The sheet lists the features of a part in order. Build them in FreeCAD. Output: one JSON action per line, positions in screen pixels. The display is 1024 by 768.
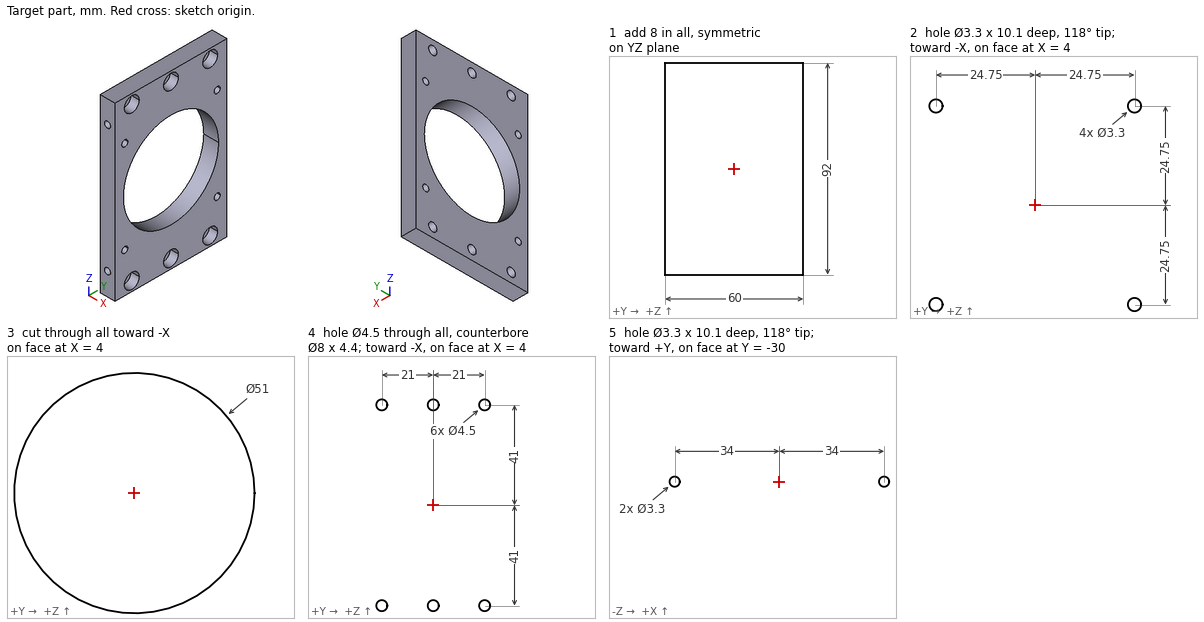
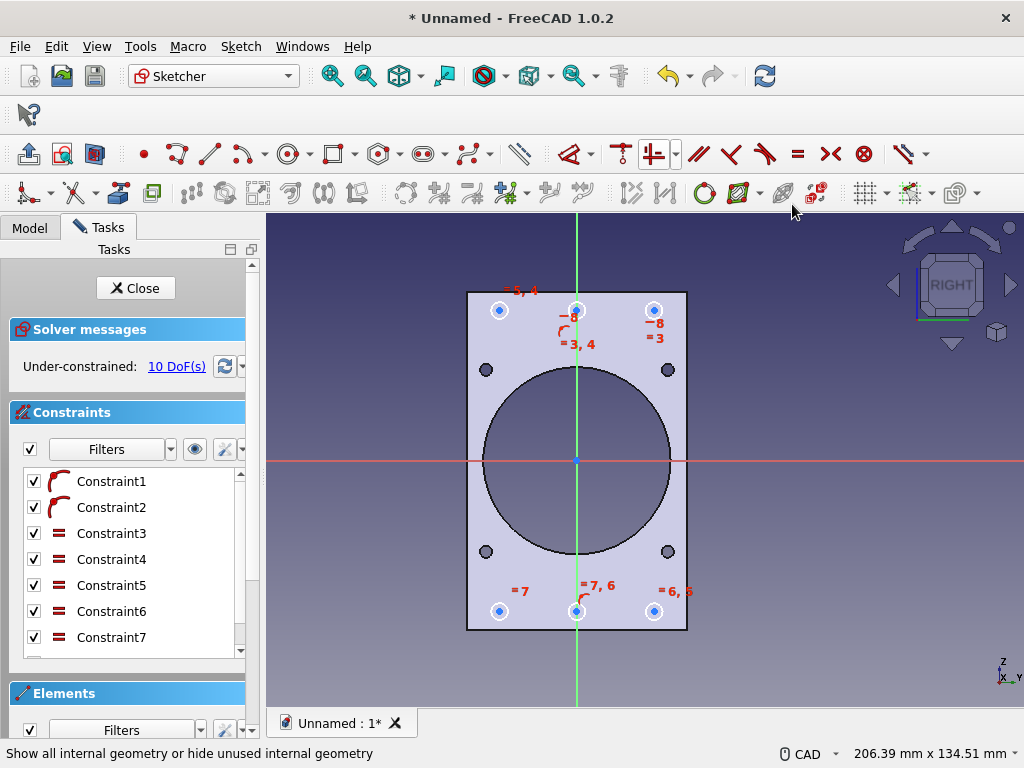
{"action": "scroll", "coordinate": [577, 311], "scroll_direction": "up", "scroll_amount": 4}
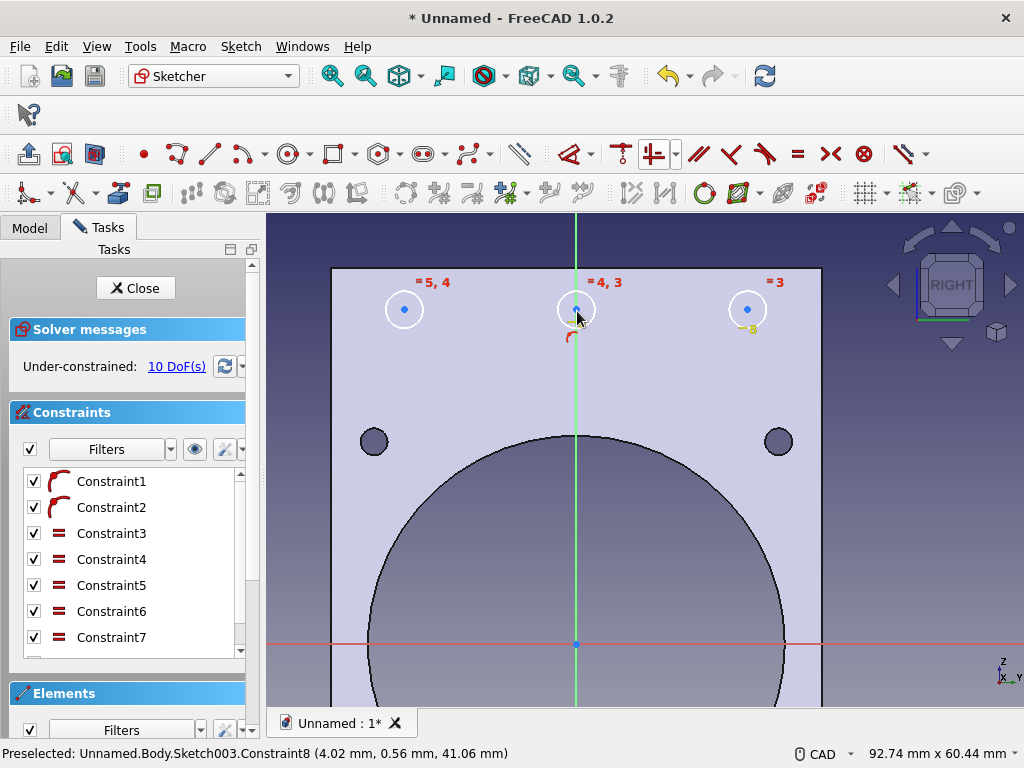
{"action": "left_click", "coordinate": [576, 310]}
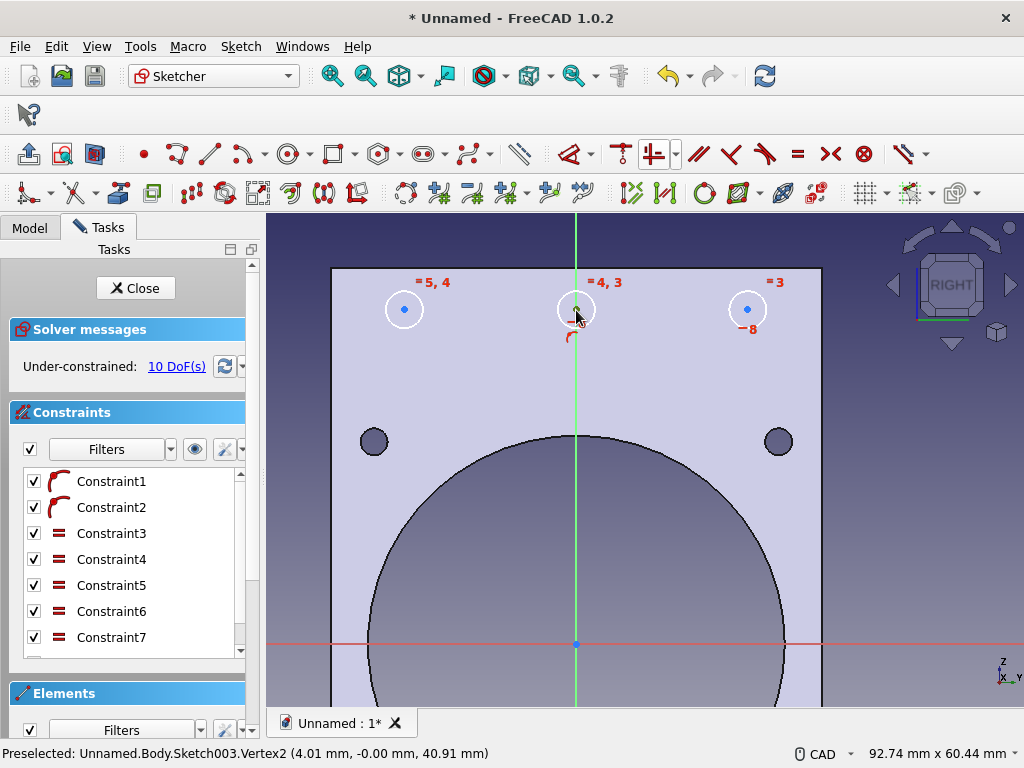
{"action": "left_click", "coordinate": [404, 310]}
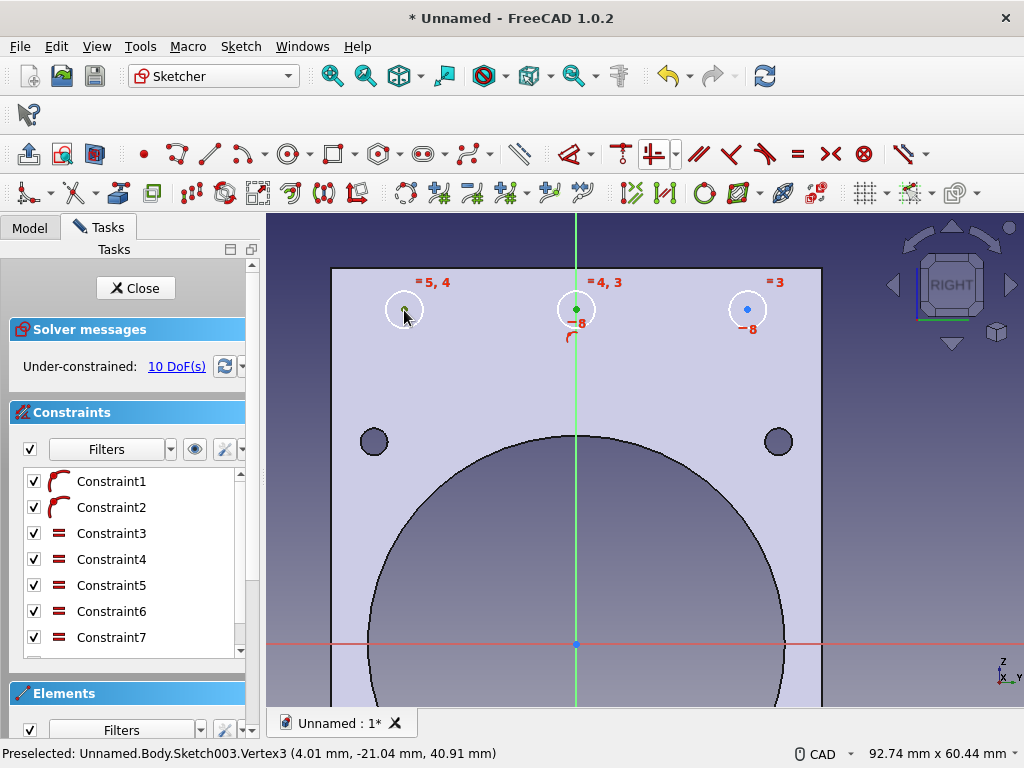
{"action": "left_click", "coordinate": [676, 154]}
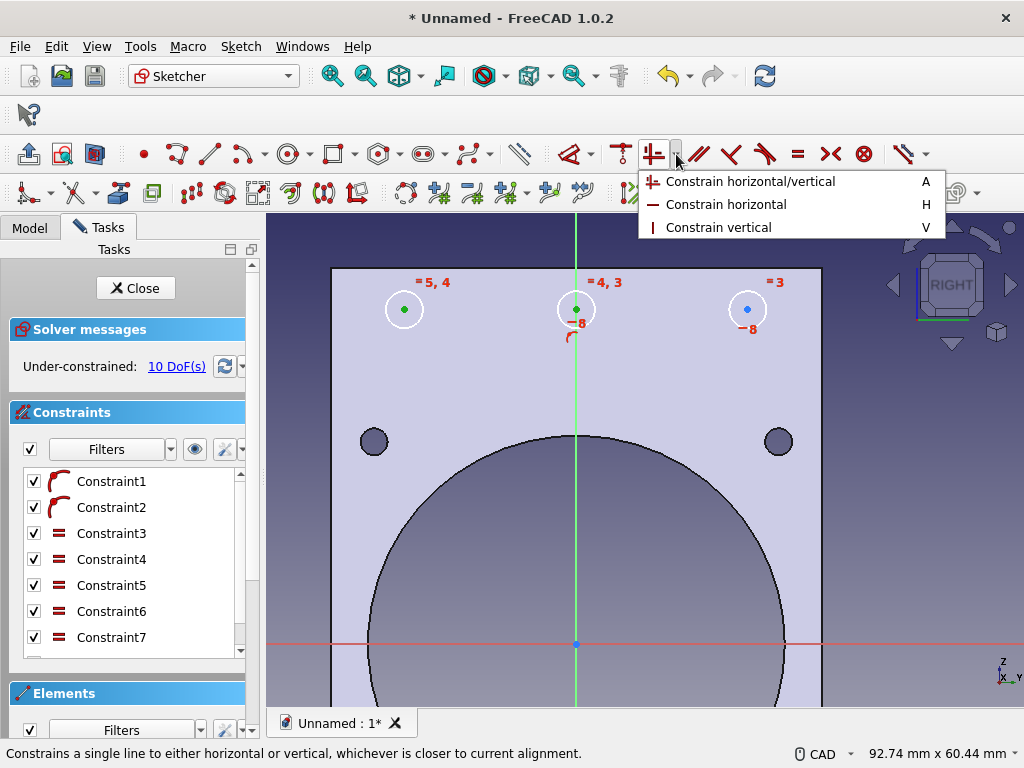
{"action": "left_click", "coordinate": [792, 204]}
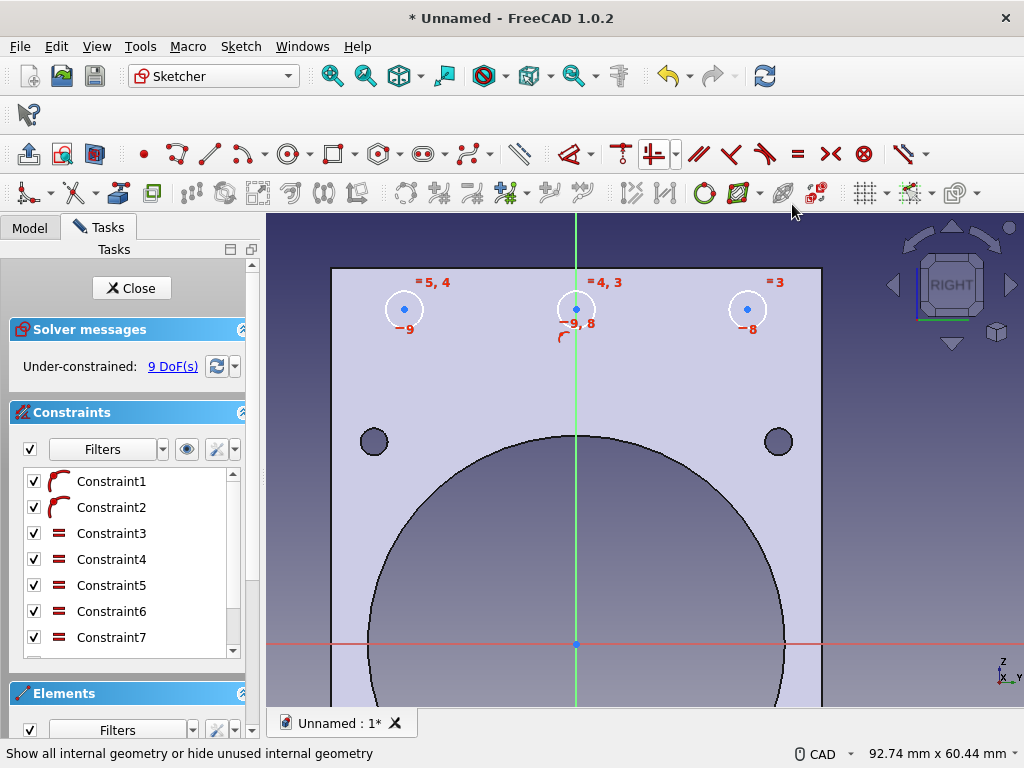
{"action": "left_click", "coordinate": [748, 310]}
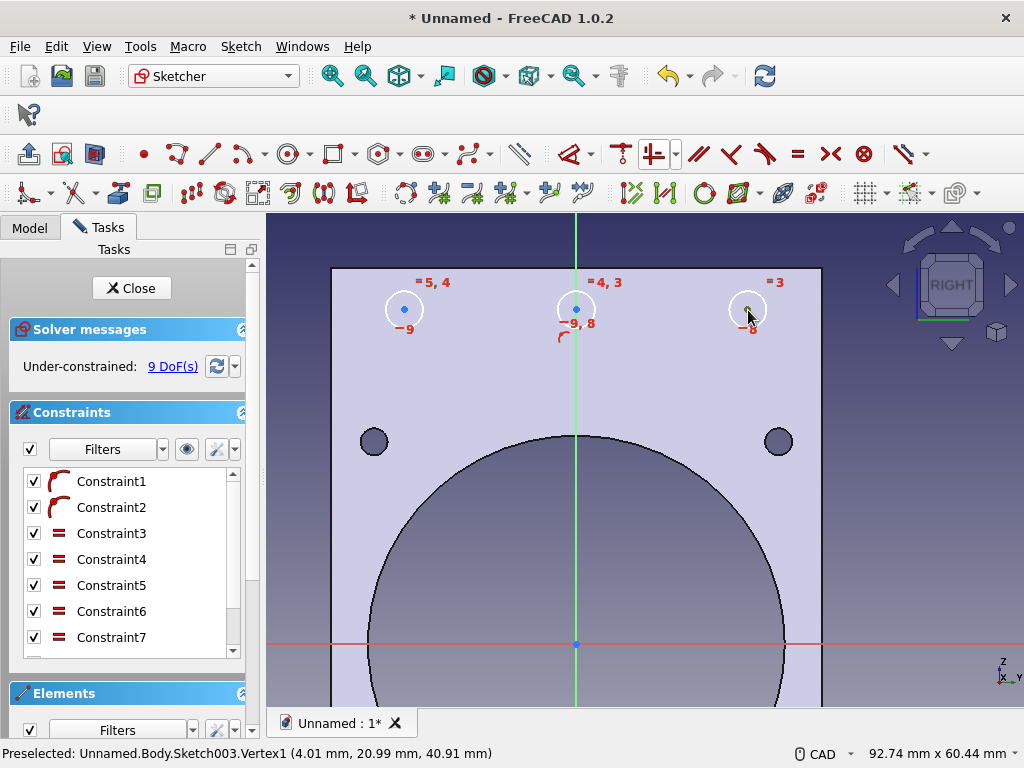
{"action": "scroll", "coordinate": [577, 310], "scroll_direction": "down", "scroll_amount": 4}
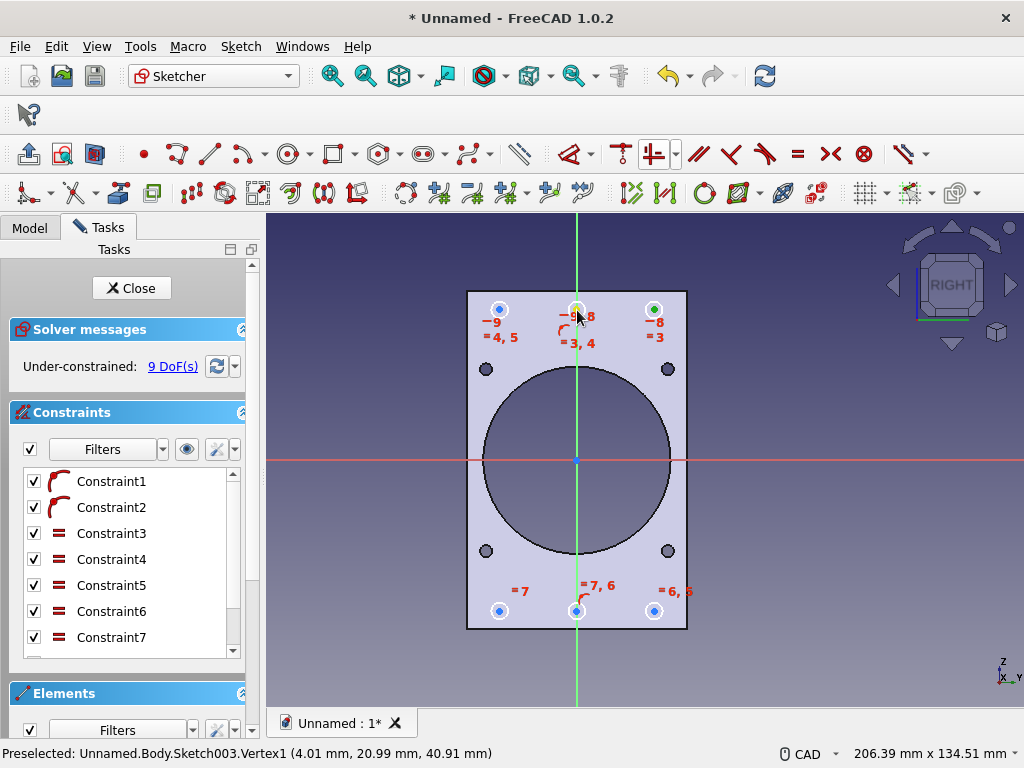
{"action": "left_click", "coordinate": [654, 611]}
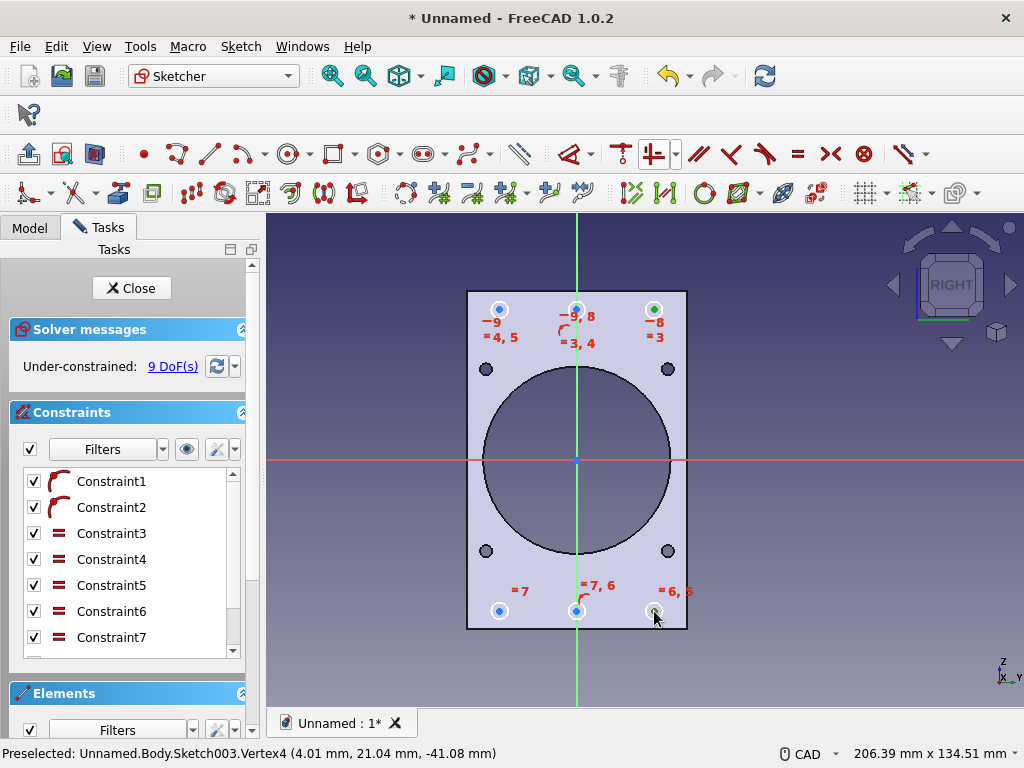
{"action": "left_click", "coordinate": [676, 154]}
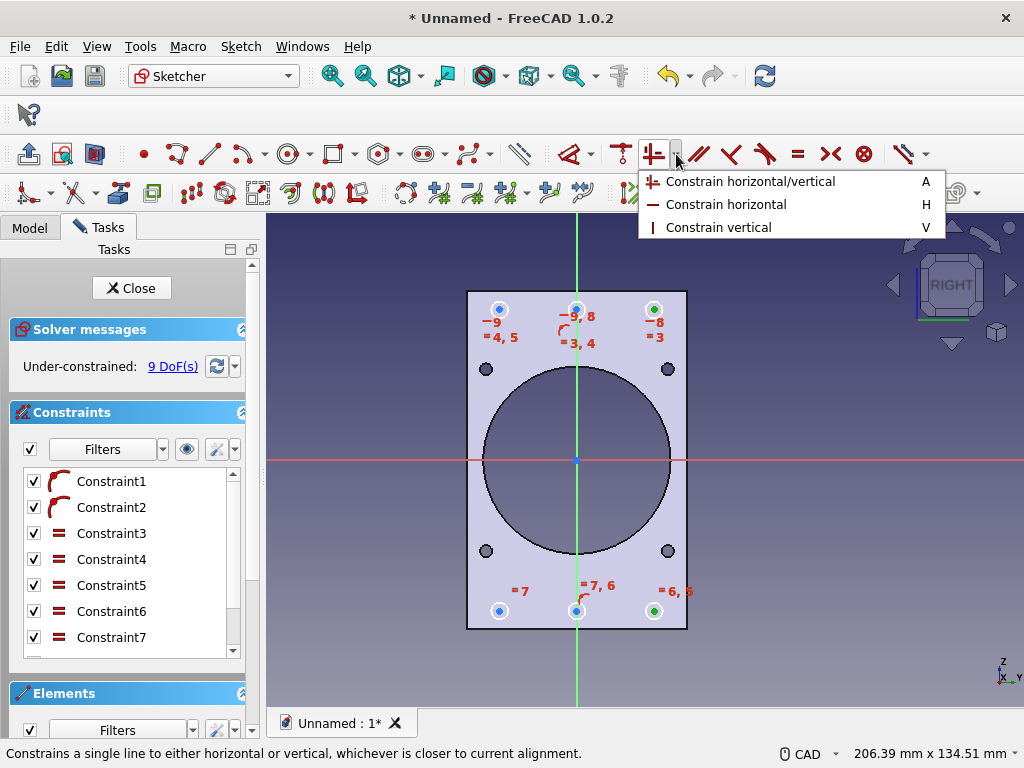
{"action": "left_click", "coordinate": [792, 228]}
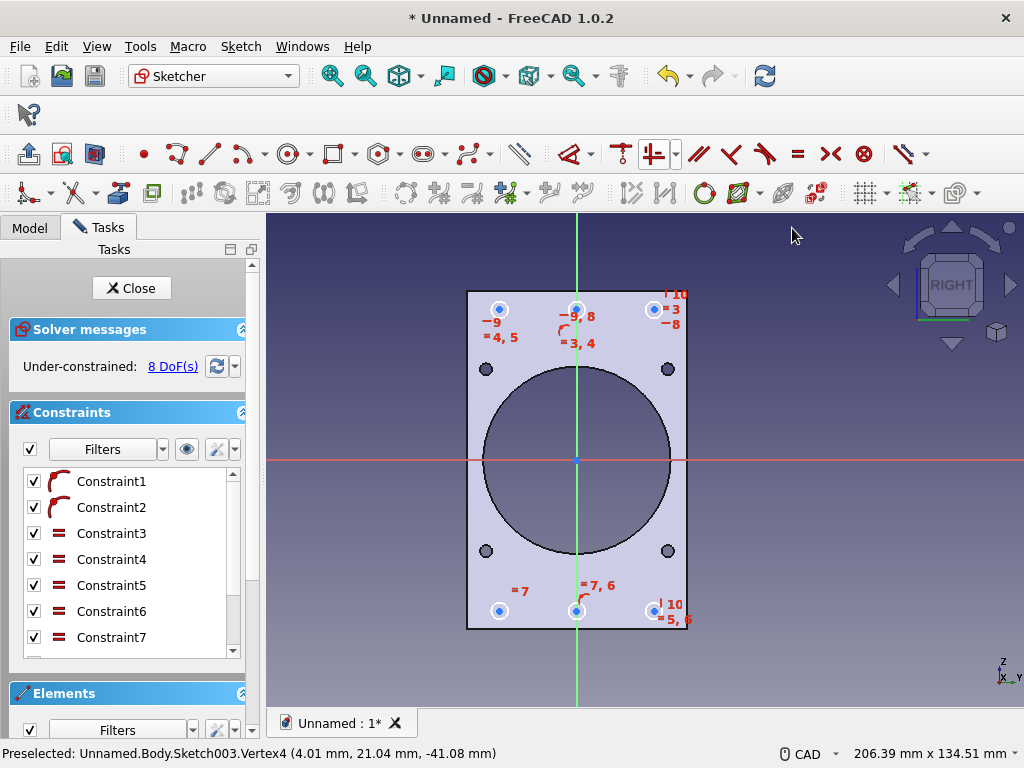
{"action": "left_click", "coordinate": [654, 611]}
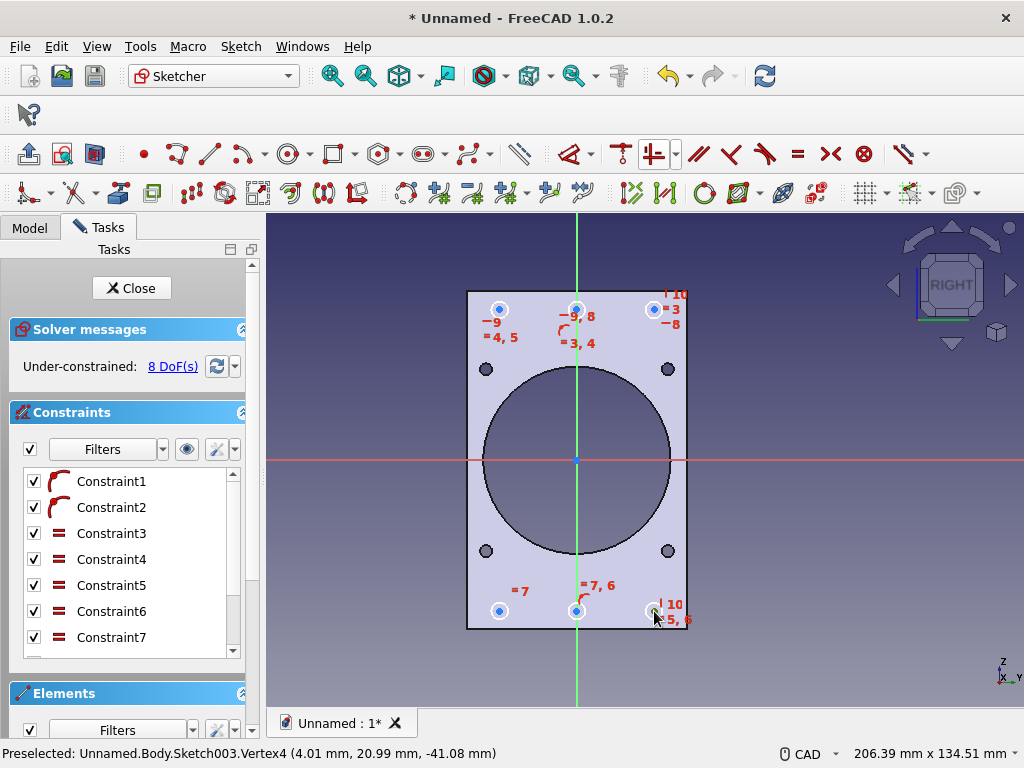
{"action": "left_click", "coordinate": [577, 611]}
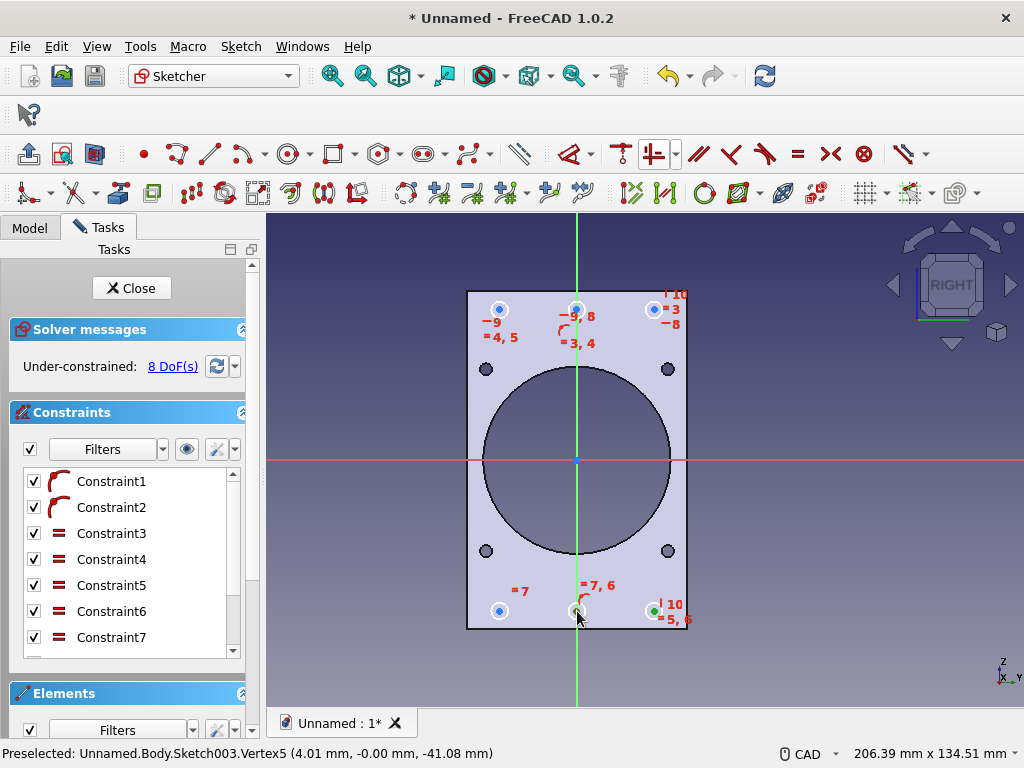
{"action": "key", "text": "h"}